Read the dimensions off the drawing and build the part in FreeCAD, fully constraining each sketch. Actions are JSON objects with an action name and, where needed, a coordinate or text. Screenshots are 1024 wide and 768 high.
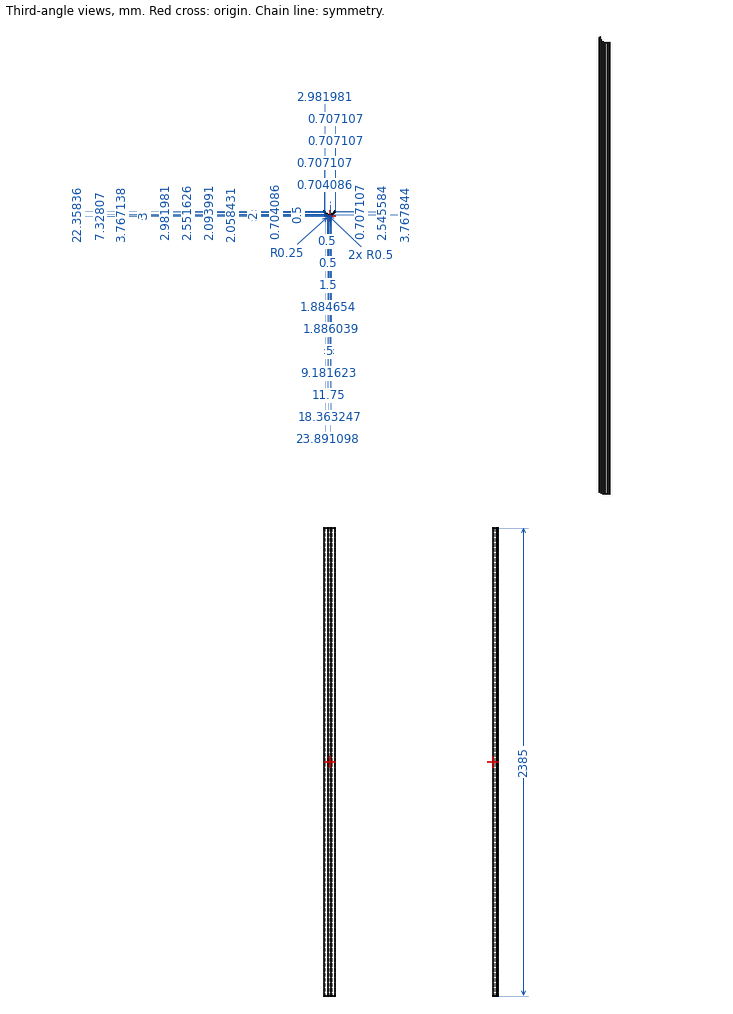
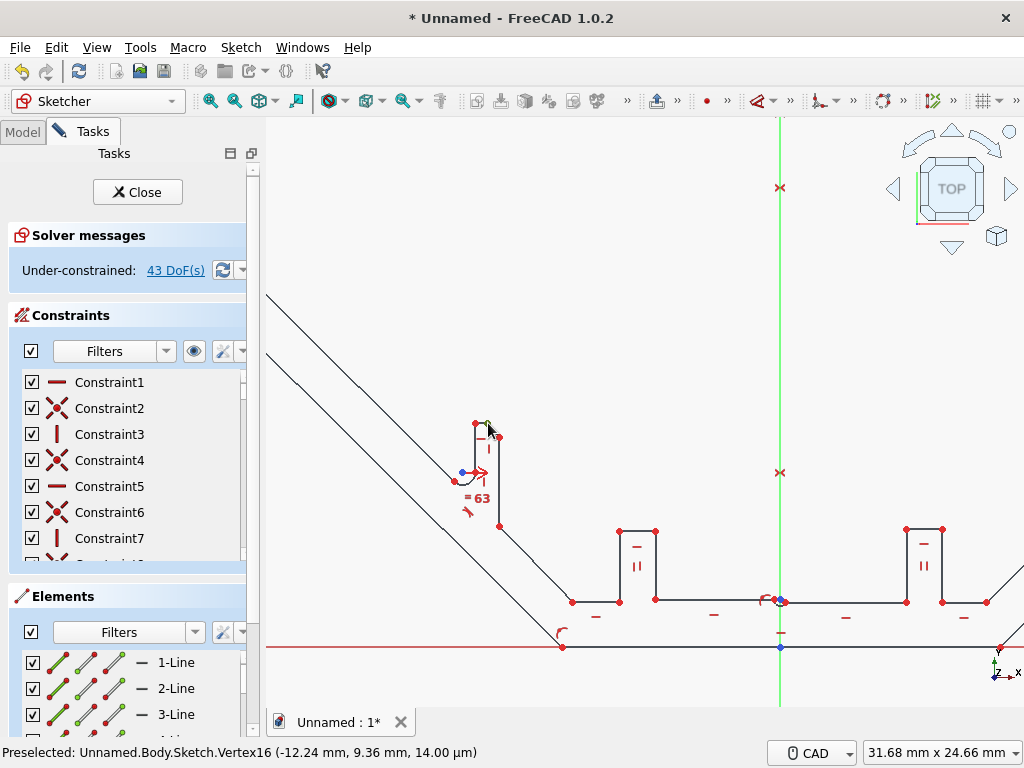
{"action": "scroll", "coordinate": [489, 426], "scroll_direction": "down", "scroll_amount": 6}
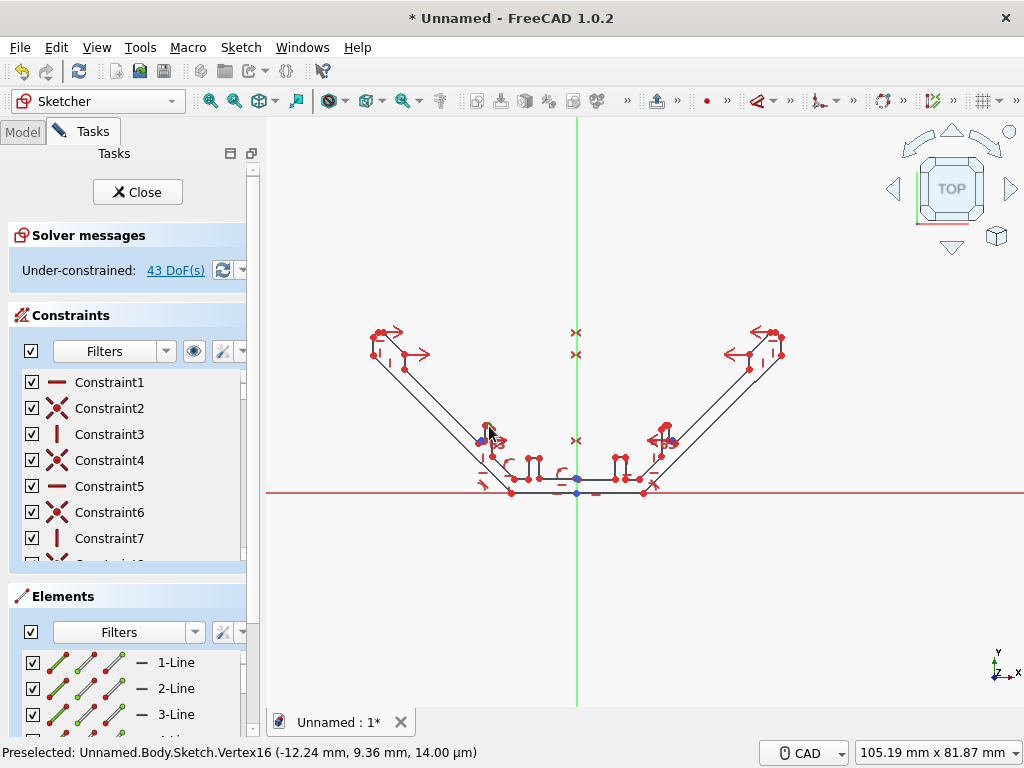
{"action": "scroll", "coordinate": [665, 426], "scroll_direction": "up", "scroll_amount": 6}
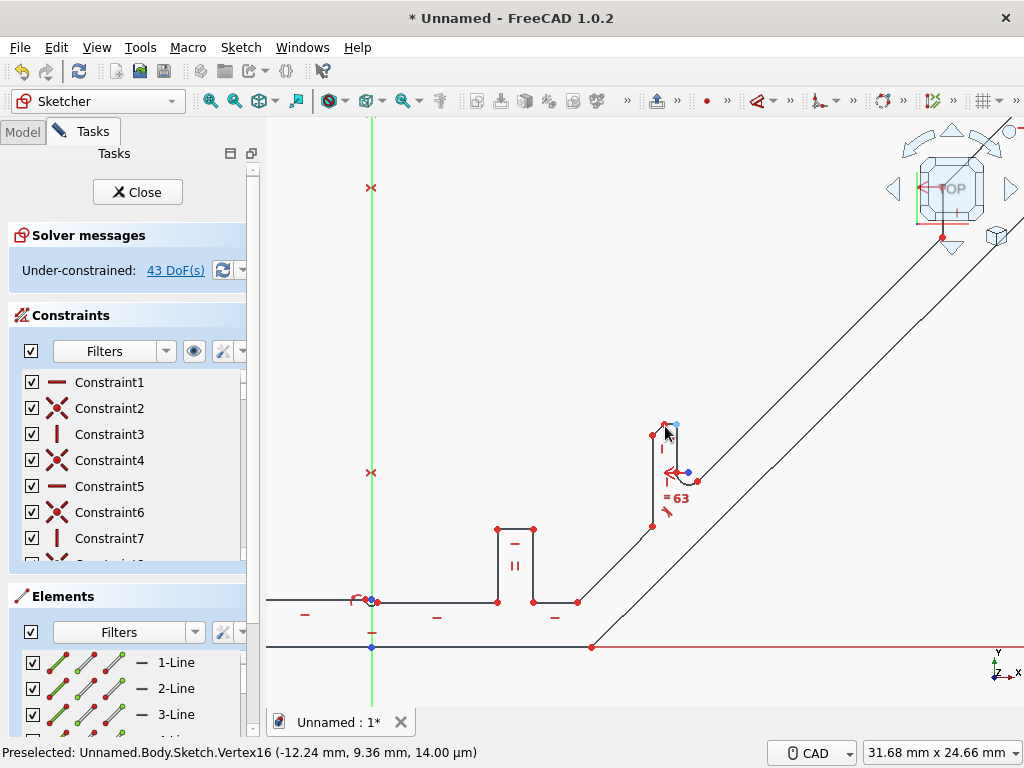
{"action": "left_click", "coordinate": [664, 424]}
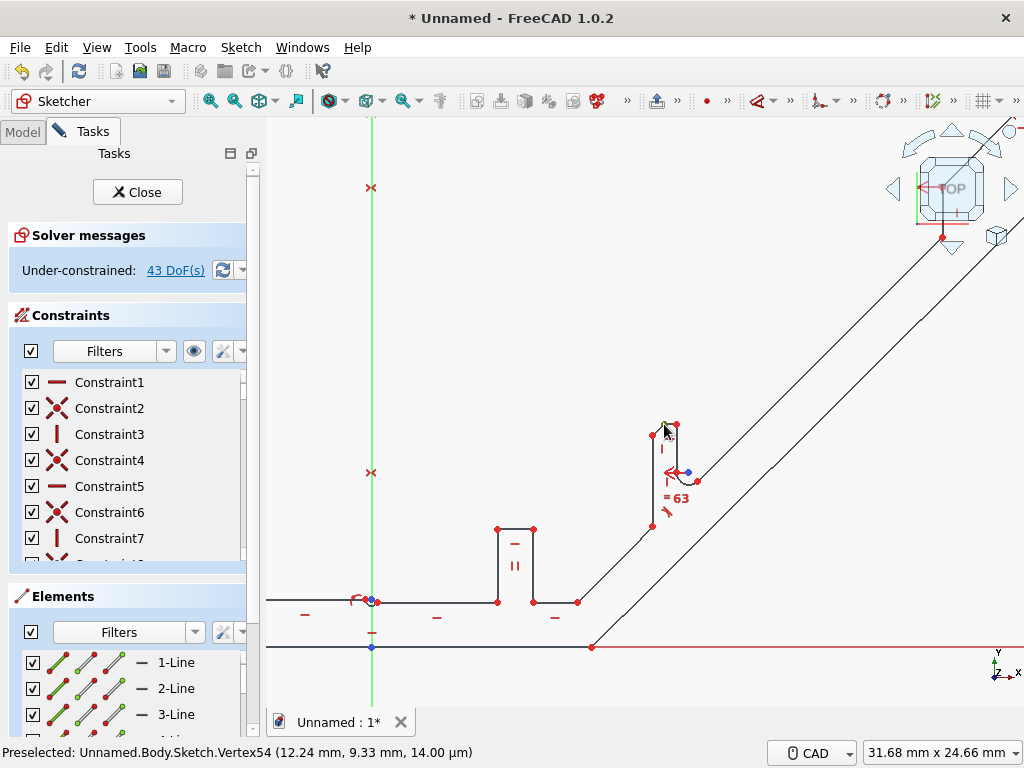
{"action": "left_click", "coordinate": [372, 565]}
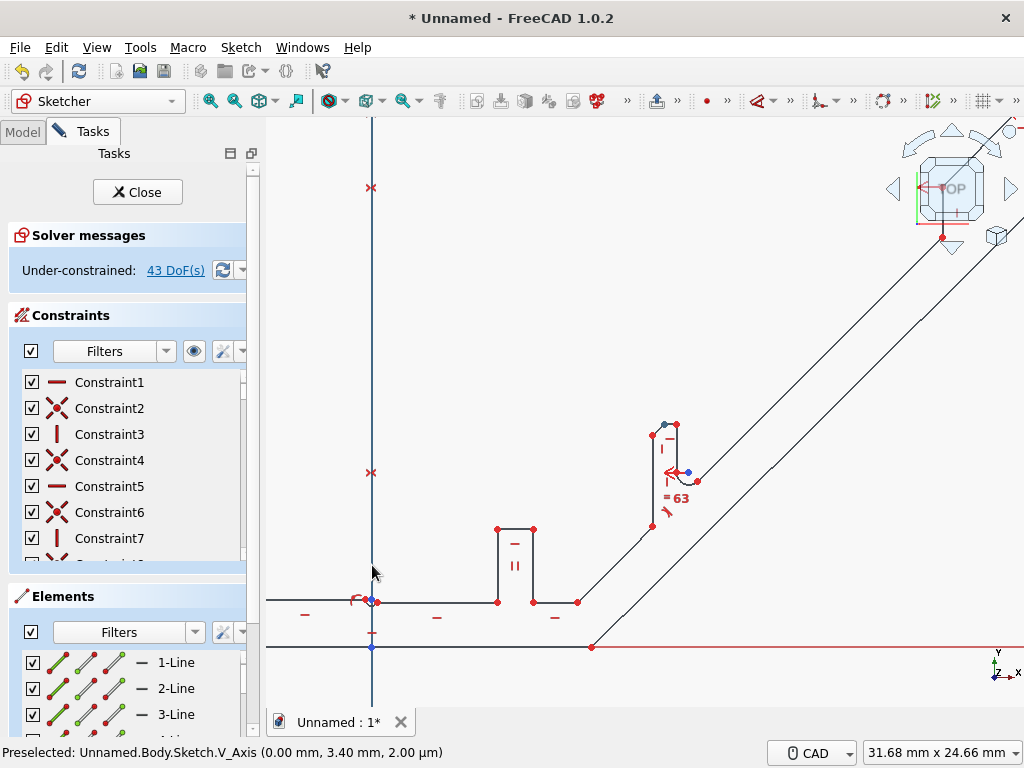
{"action": "key", "text": "s"}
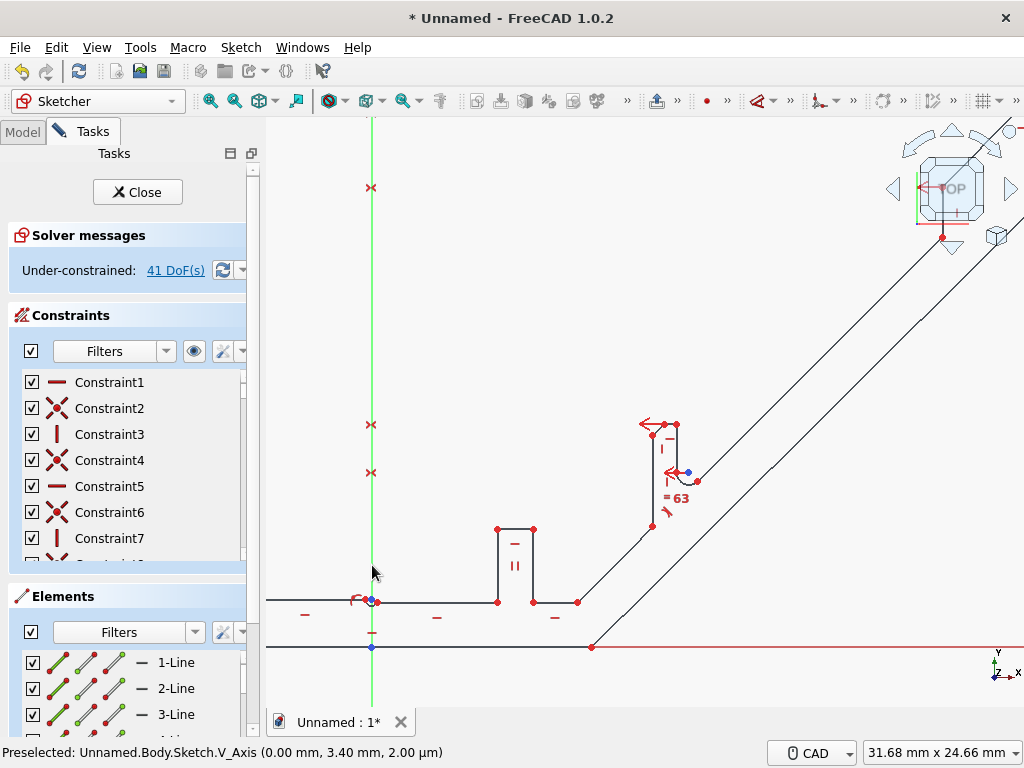
{"action": "scroll", "coordinate": [665, 426], "scroll_direction": "down", "scroll_amount": 6}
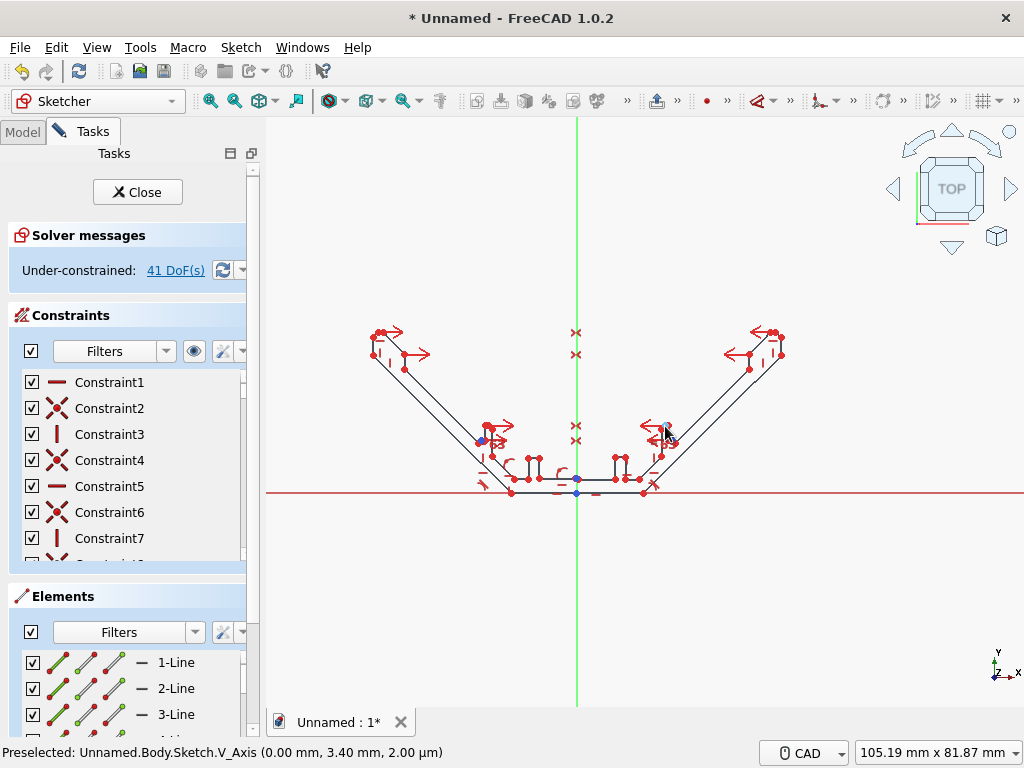
{"action": "scroll", "coordinate": [492, 430], "scroll_direction": "up", "scroll_amount": 5}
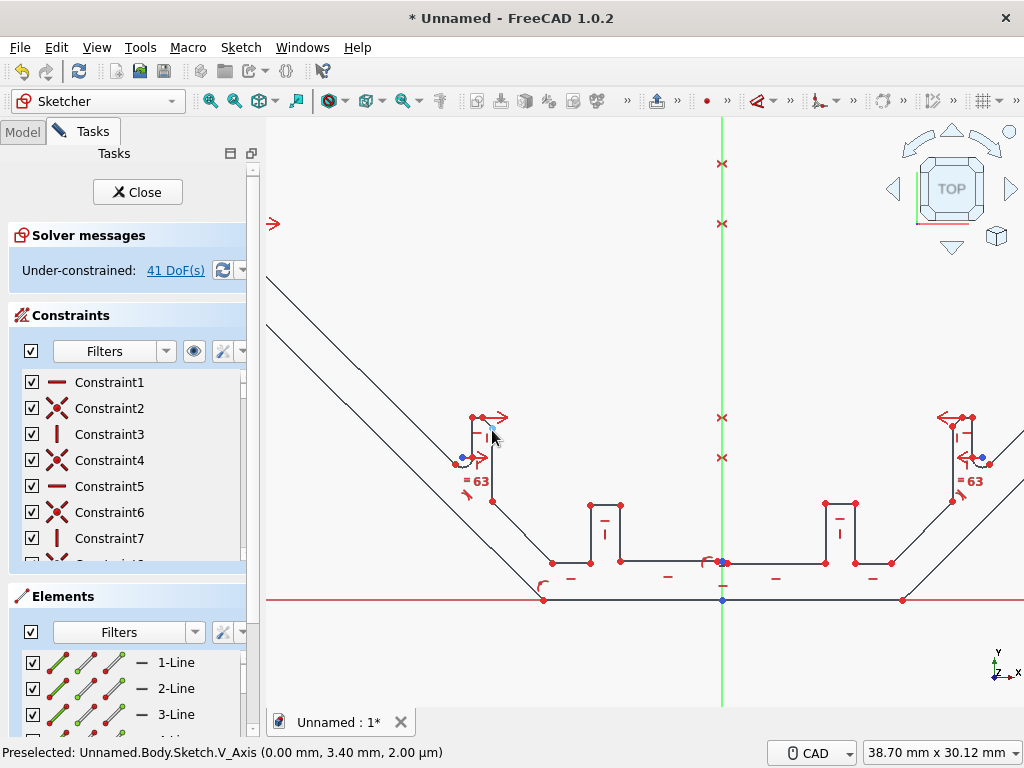
{"action": "left_click", "coordinate": [492, 429]}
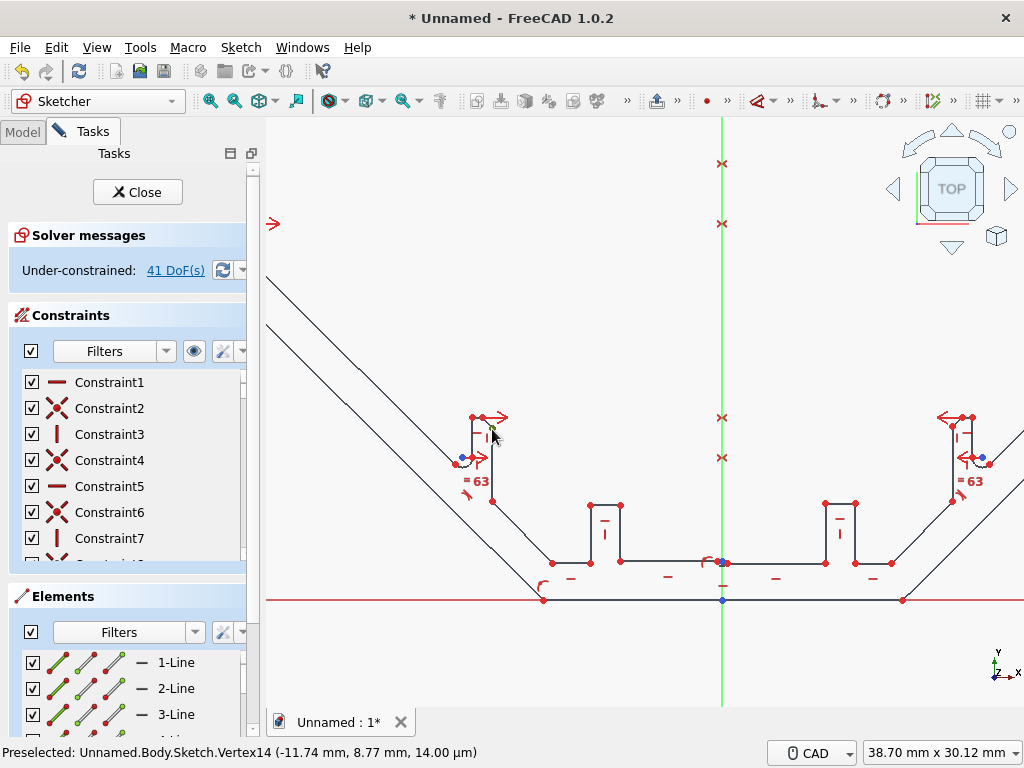
{"action": "scroll", "coordinate": [492, 430], "scroll_direction": "down", "scroll_amount": 5}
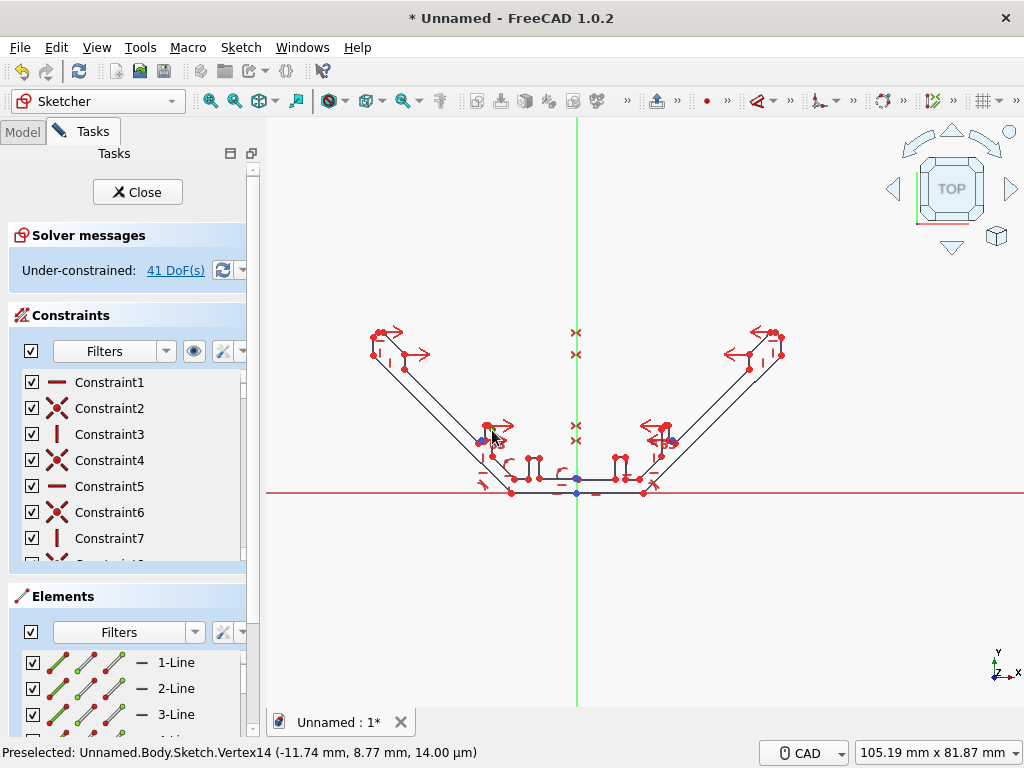
{"action": "scroll", "coordinate": [662, 429], "scroll_direction": "up", "scroll_amount": 5}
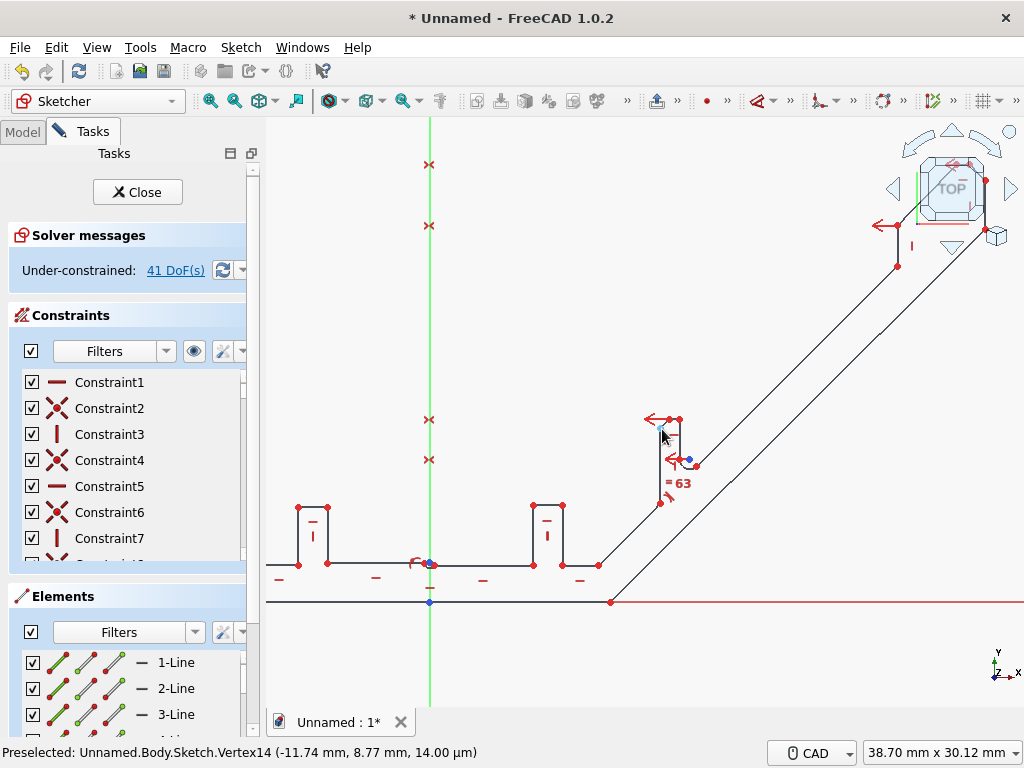
{"action": "left_click", "coordinate": [660, 428]}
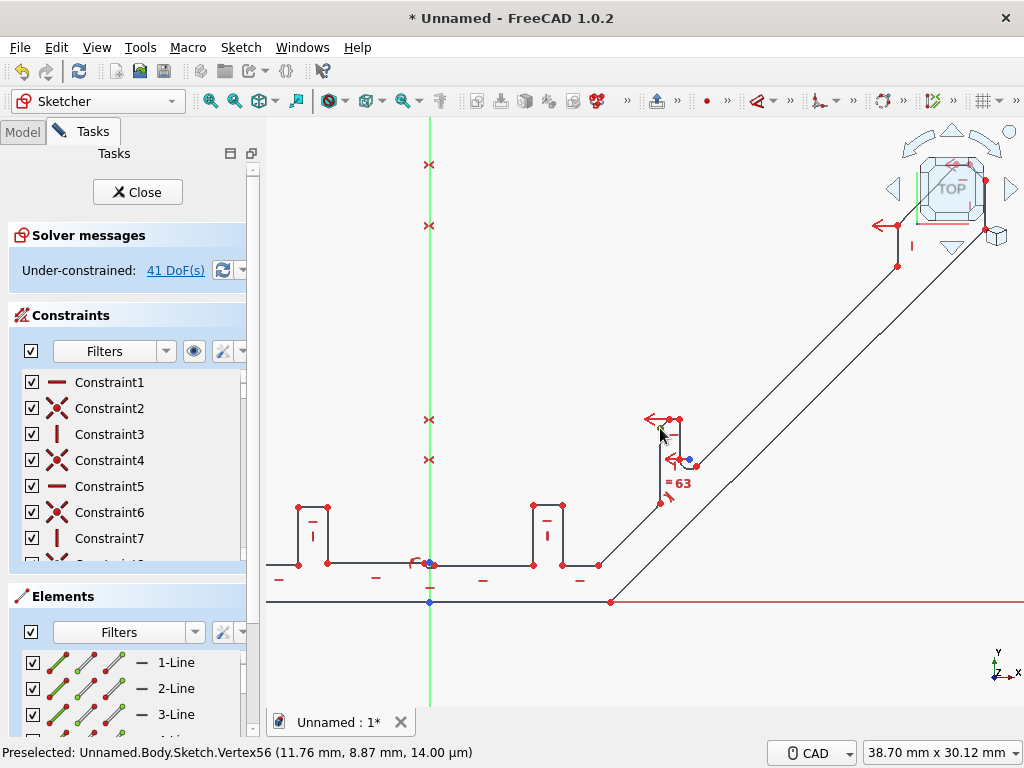
{"action": "left_click", "coordinate": [430, 641]}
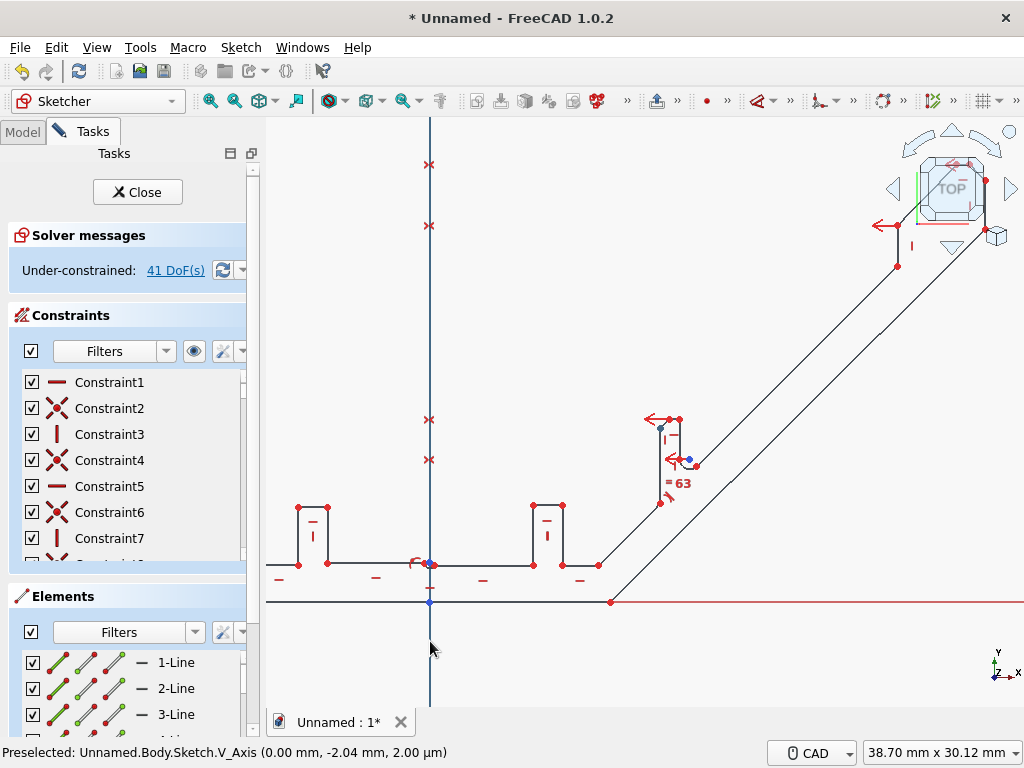
{"action": "key", "text": "s"}